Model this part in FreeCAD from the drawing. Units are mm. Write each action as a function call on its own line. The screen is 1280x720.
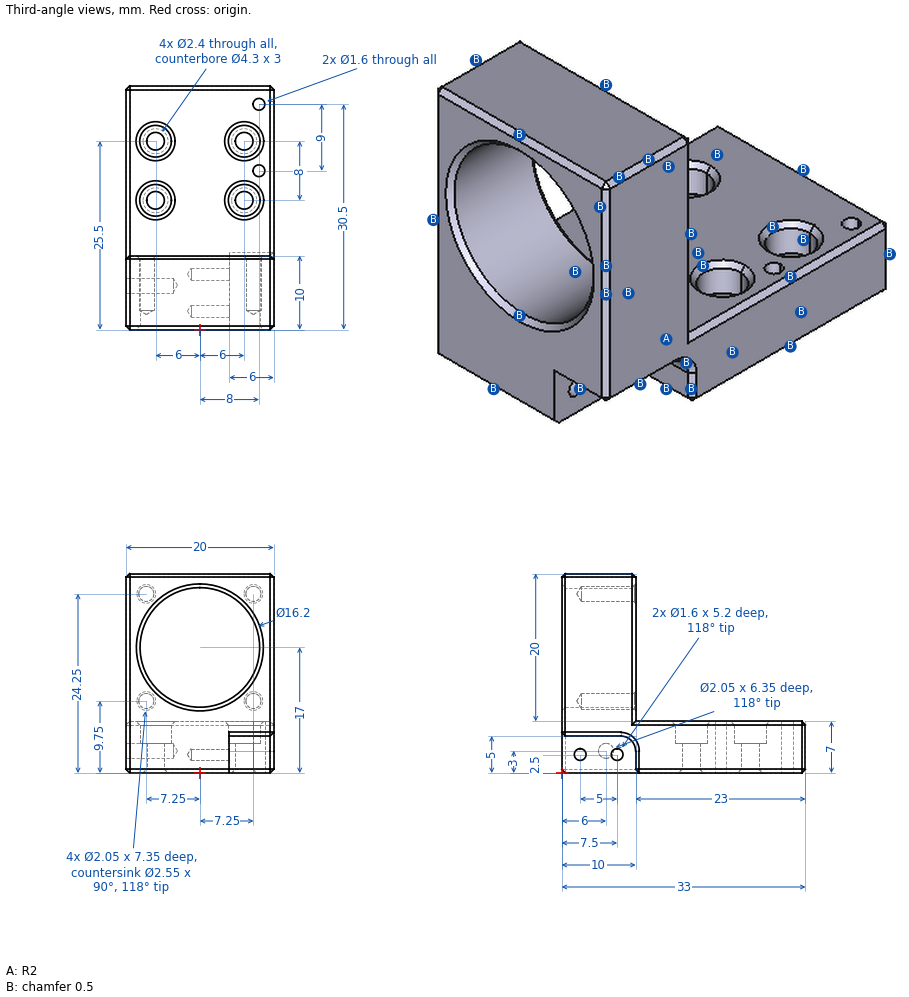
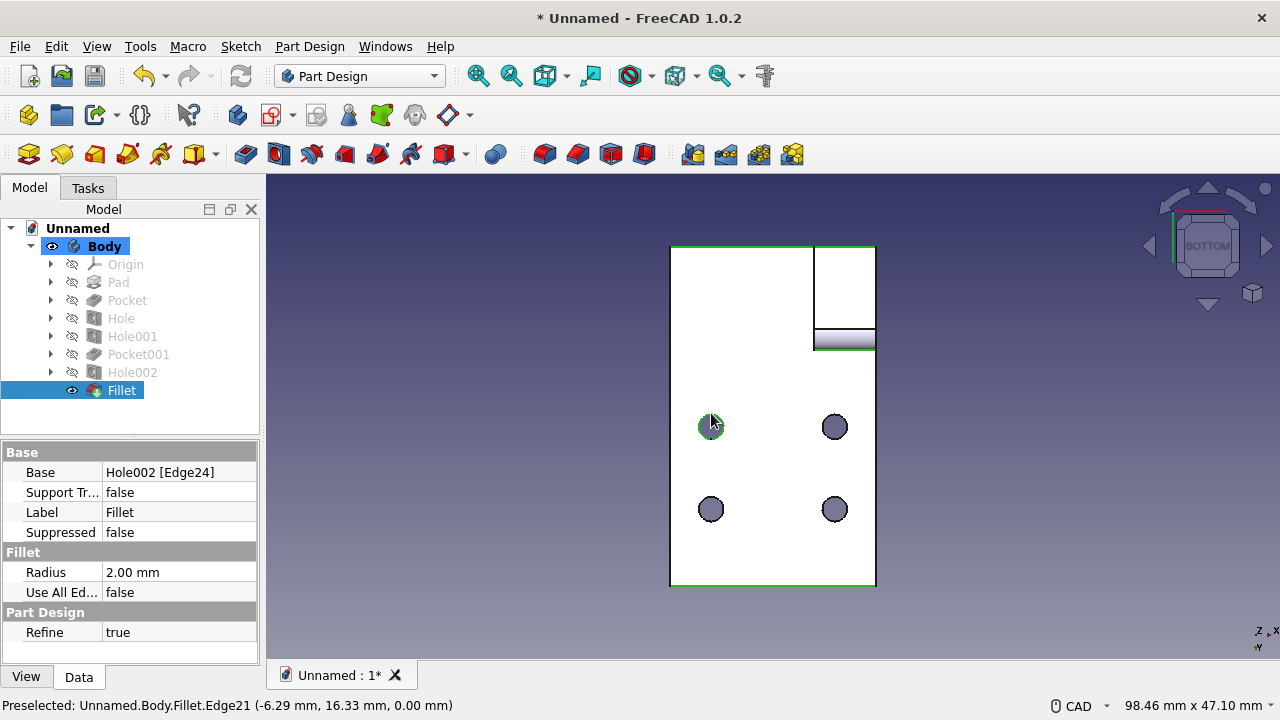
click(835, 413, ctrl)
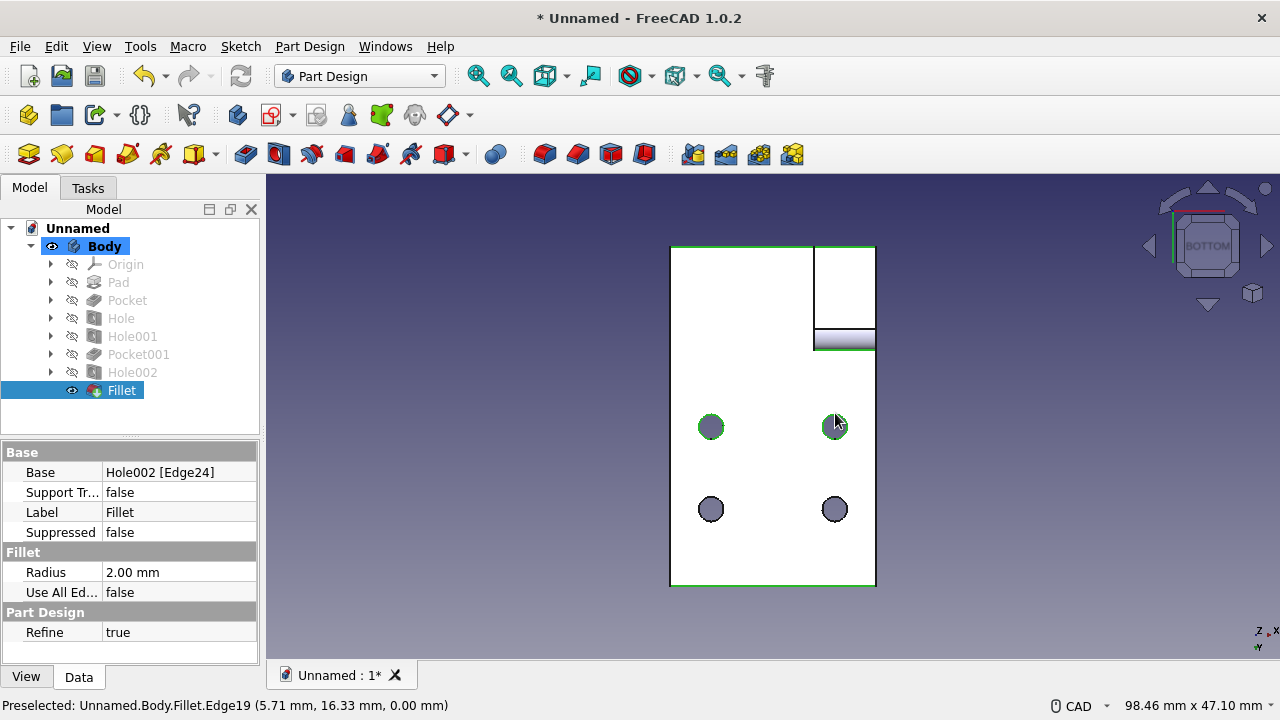
click(842, 498, ctrl)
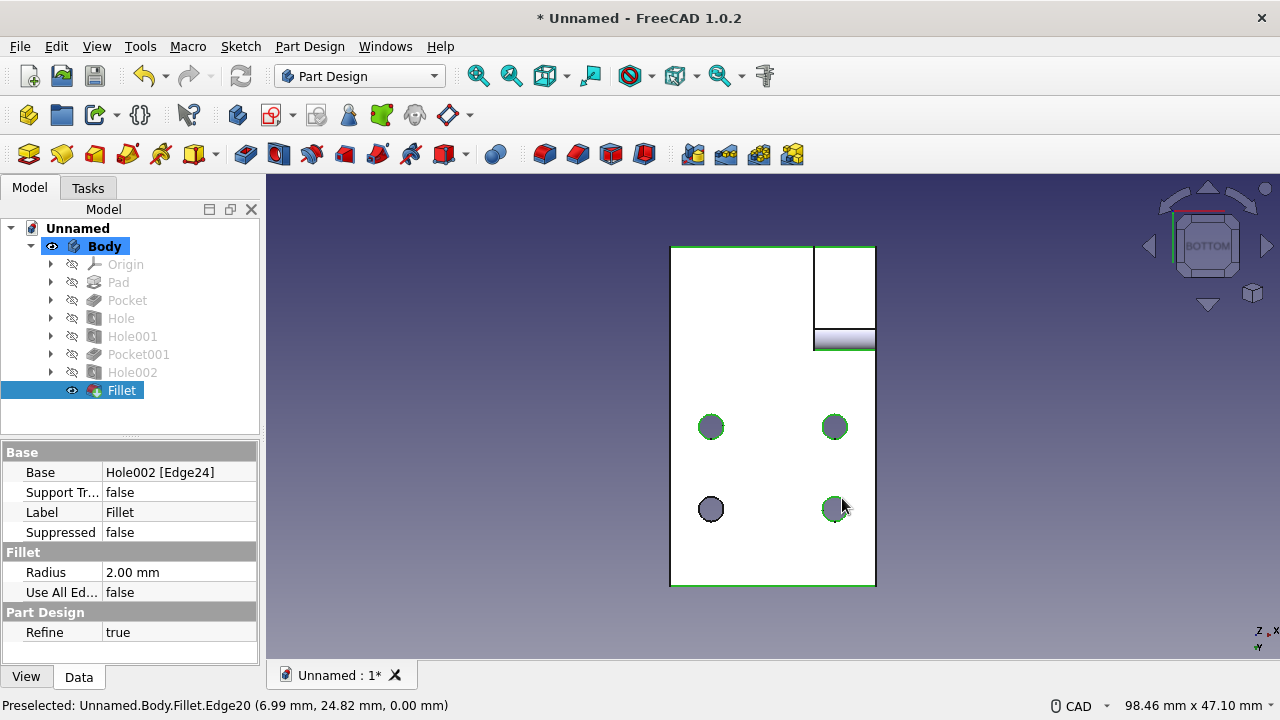
click(718, 498, ctrl)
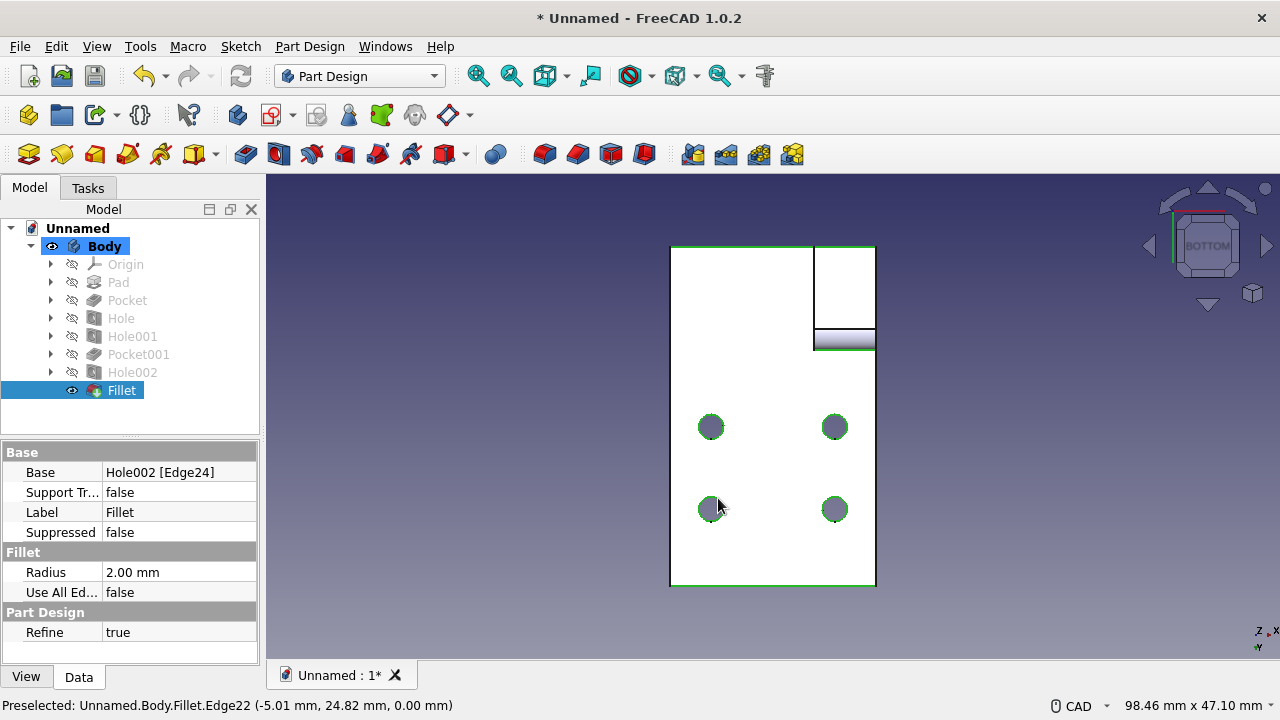
key(4)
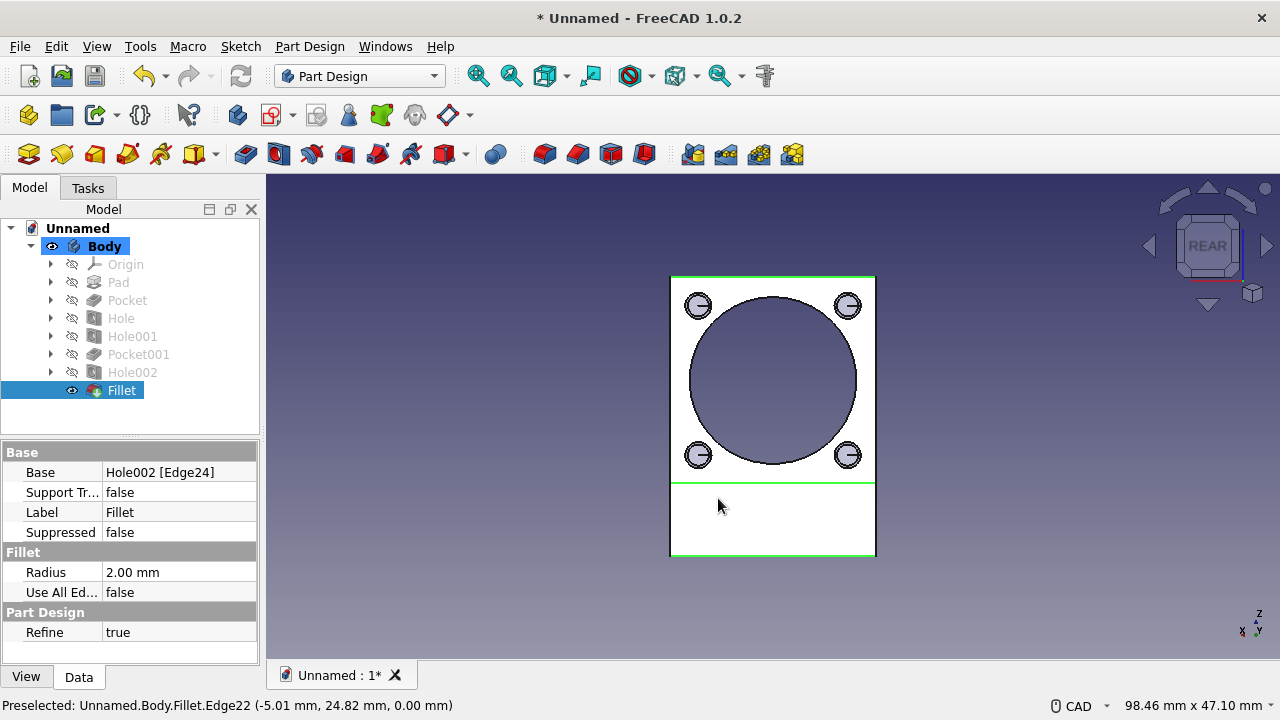
click(773, 463, ctrl)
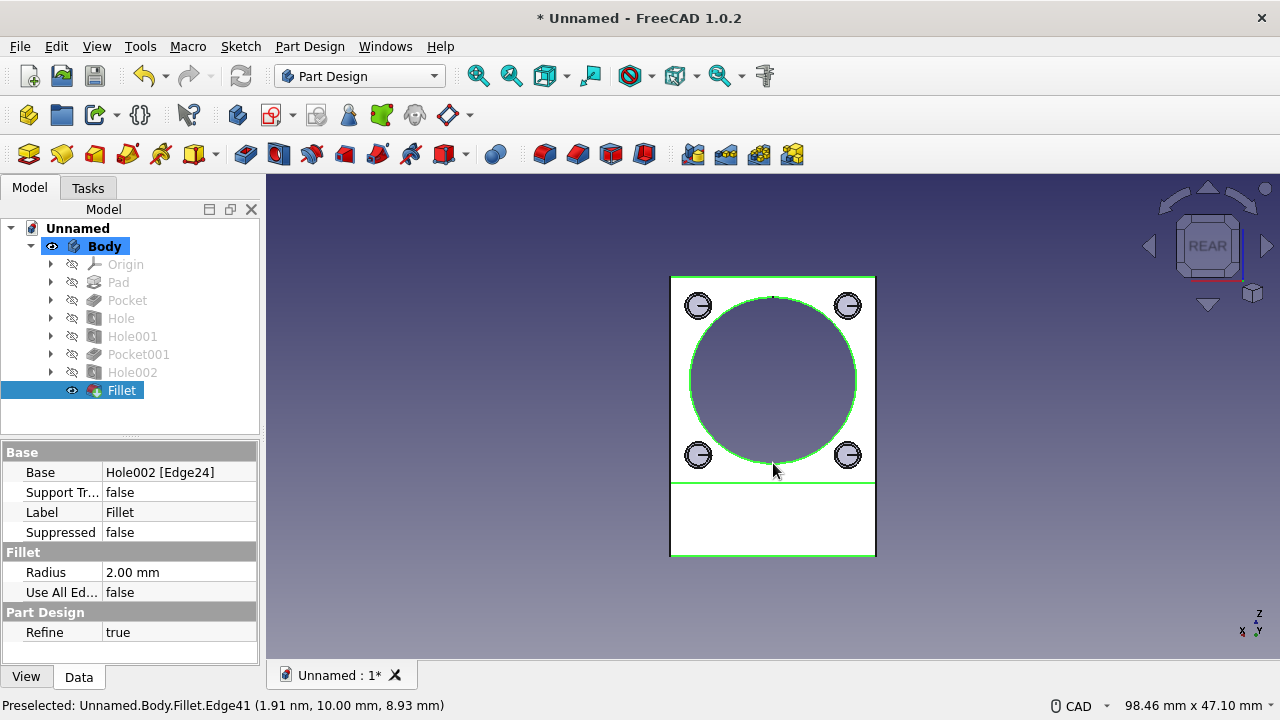
key(6)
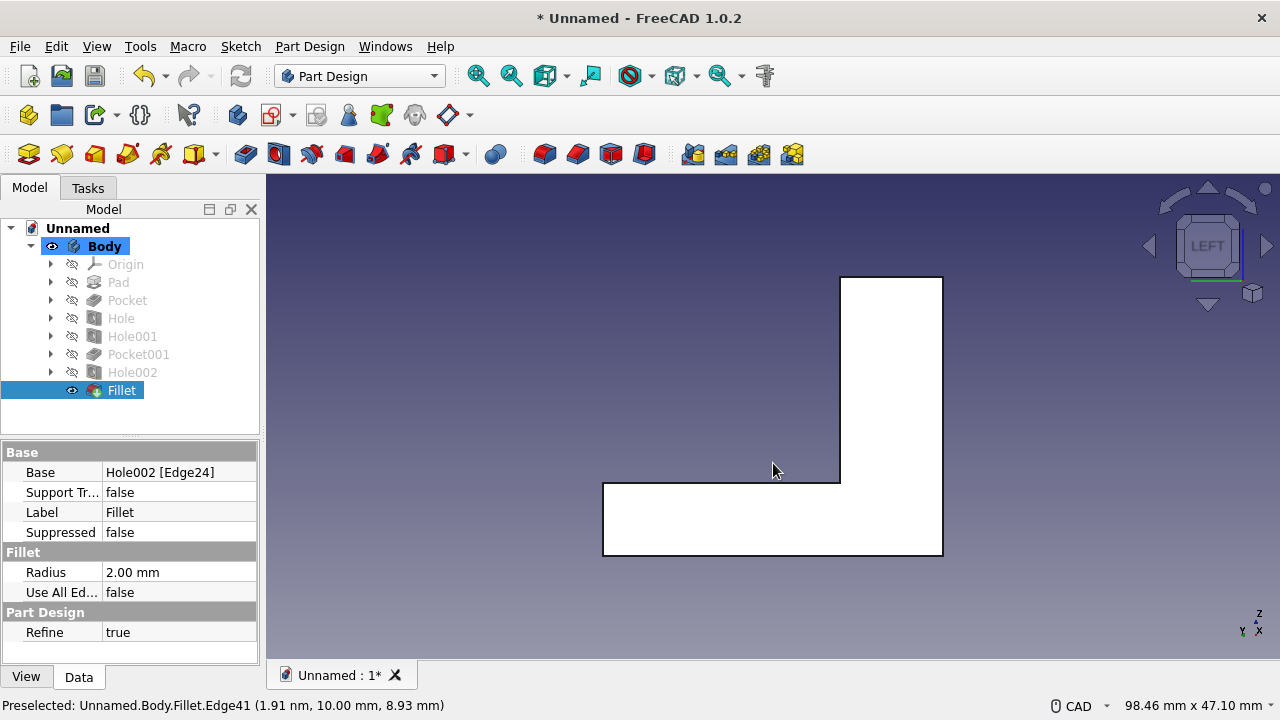
click(870, 495, ctrl)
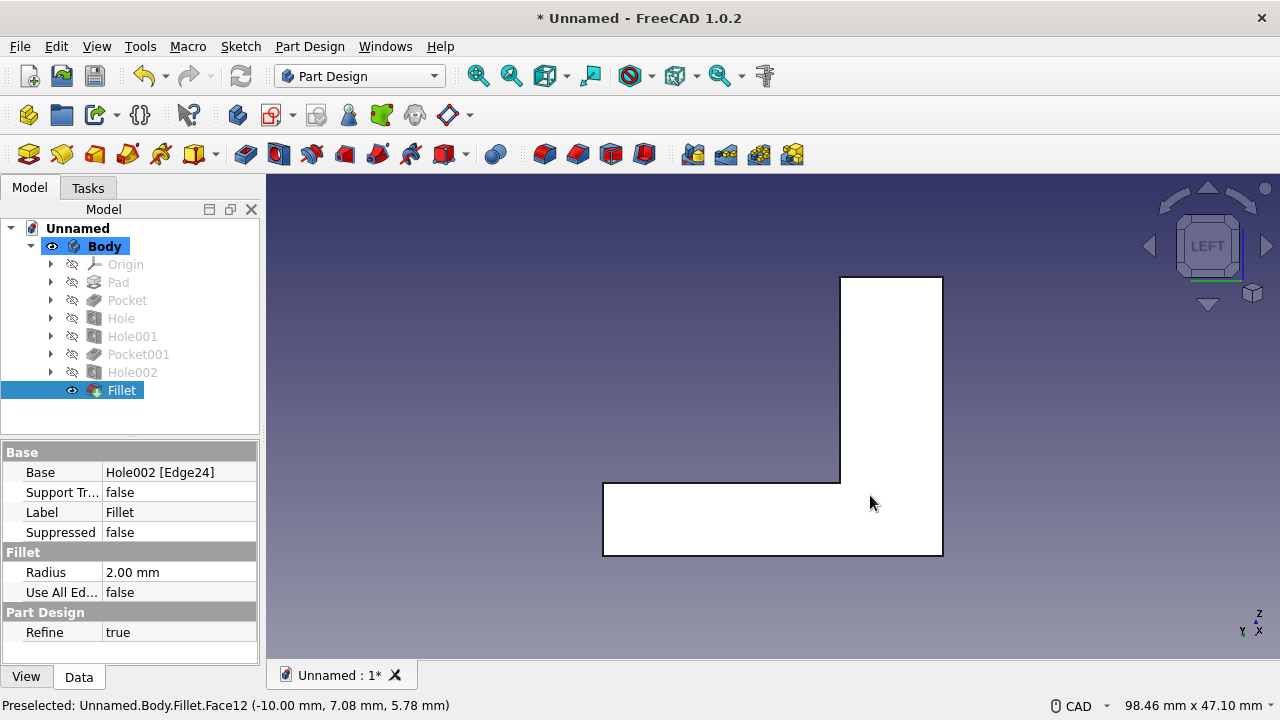
click(578, 154)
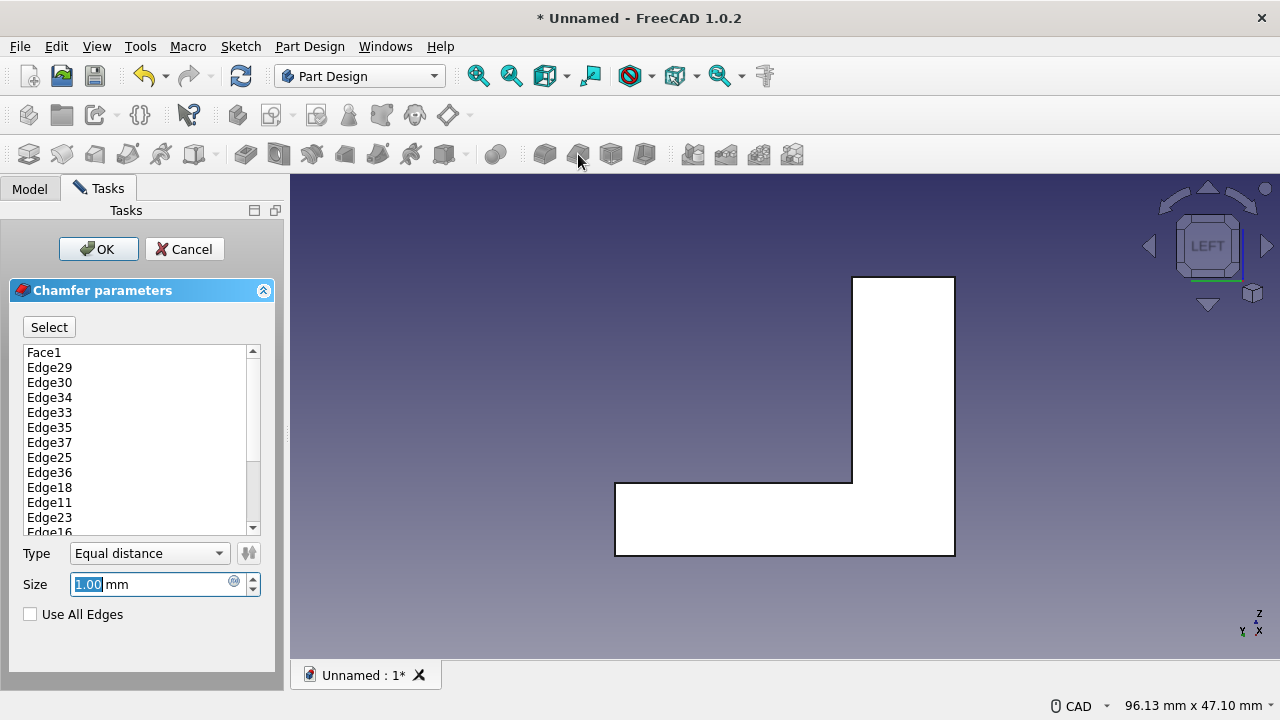
text(0.5)
key(Tab)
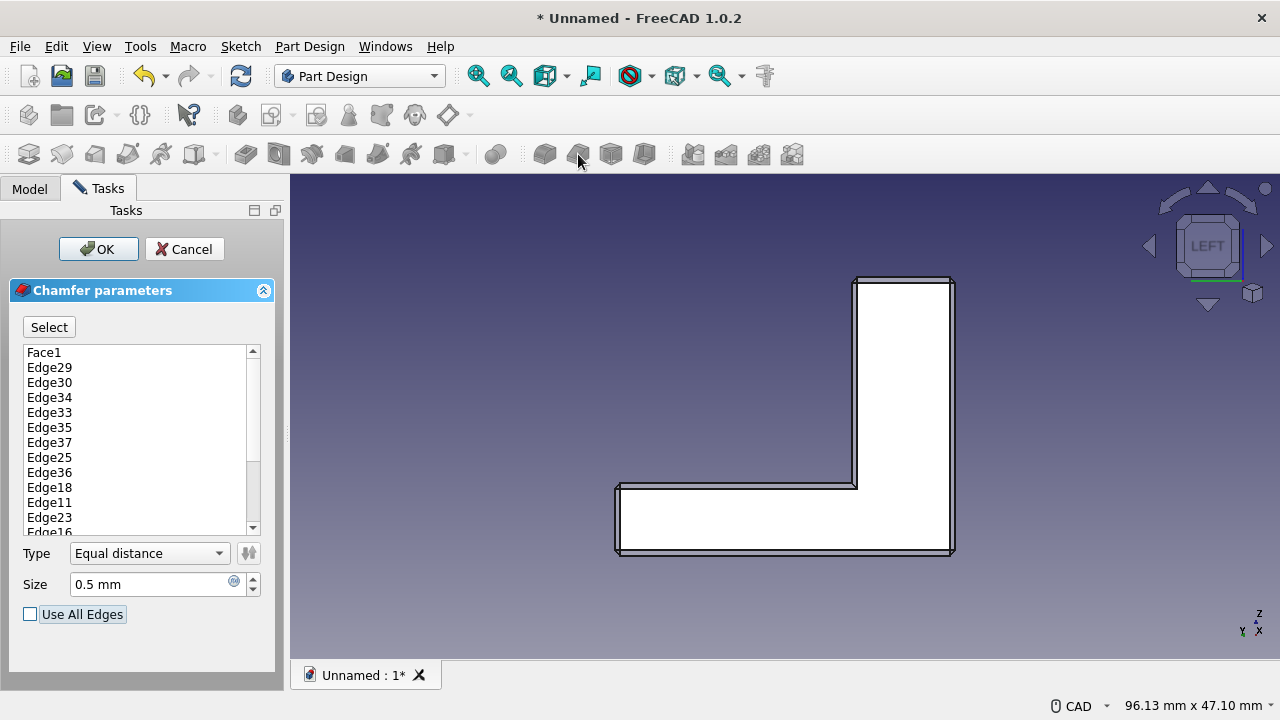
click(99, 249)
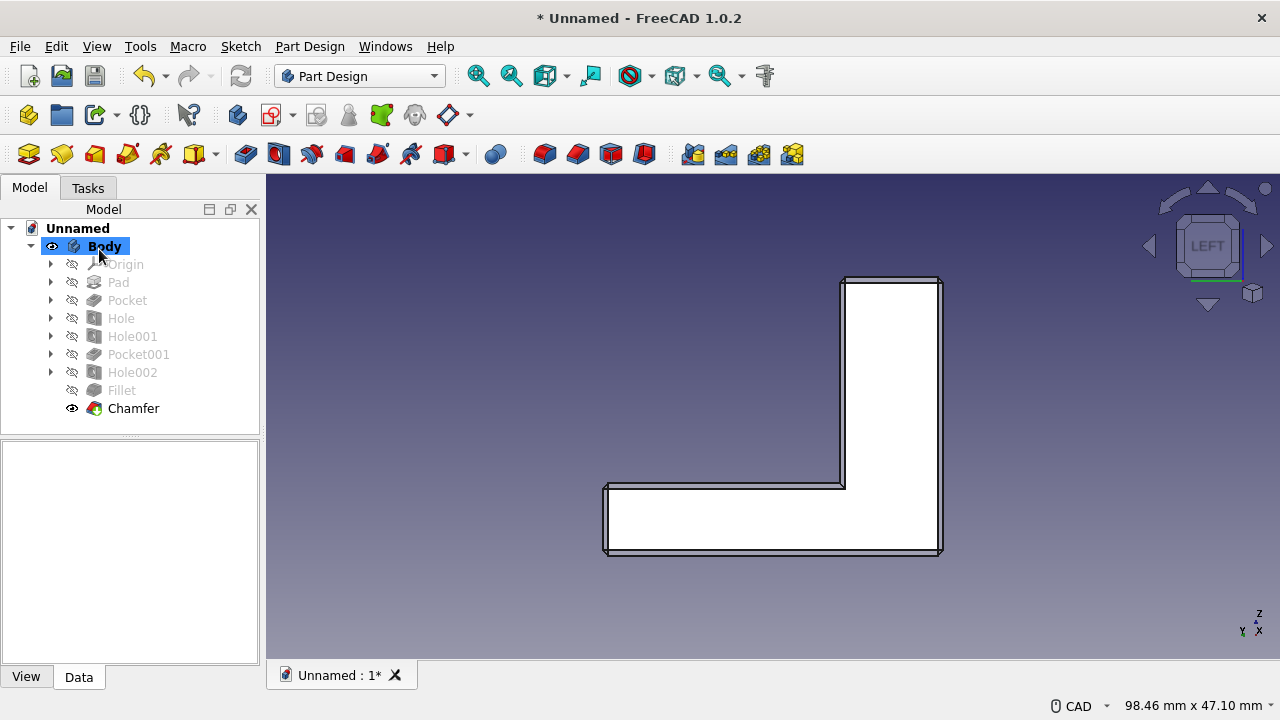
click(914, 454)